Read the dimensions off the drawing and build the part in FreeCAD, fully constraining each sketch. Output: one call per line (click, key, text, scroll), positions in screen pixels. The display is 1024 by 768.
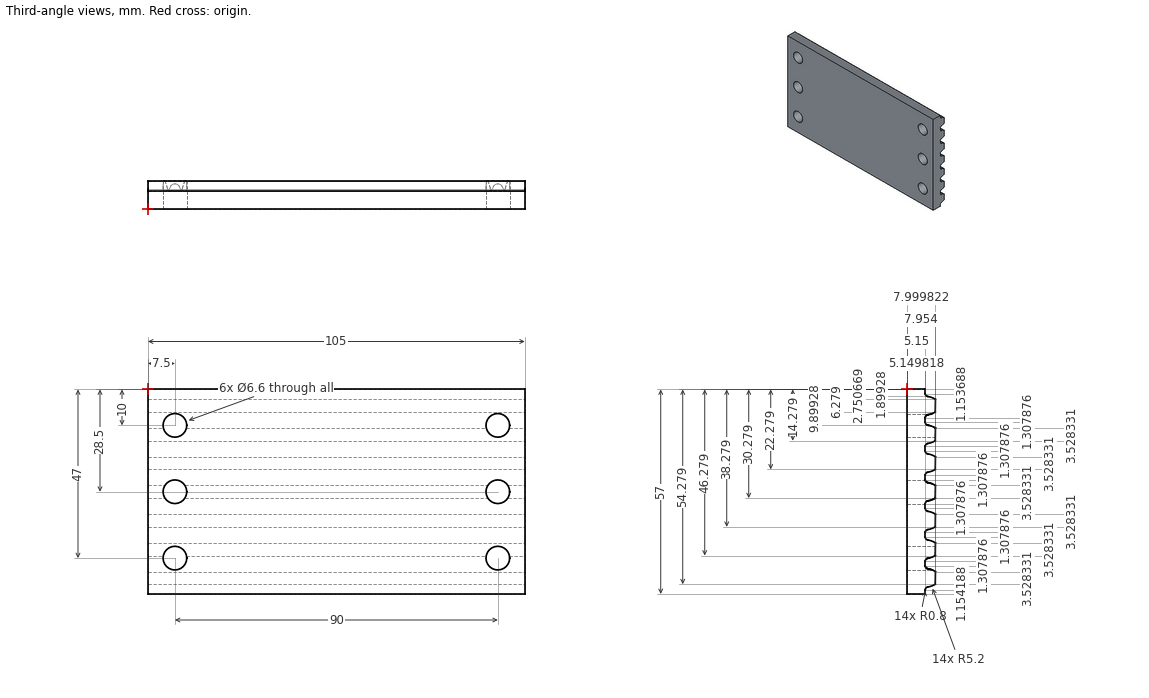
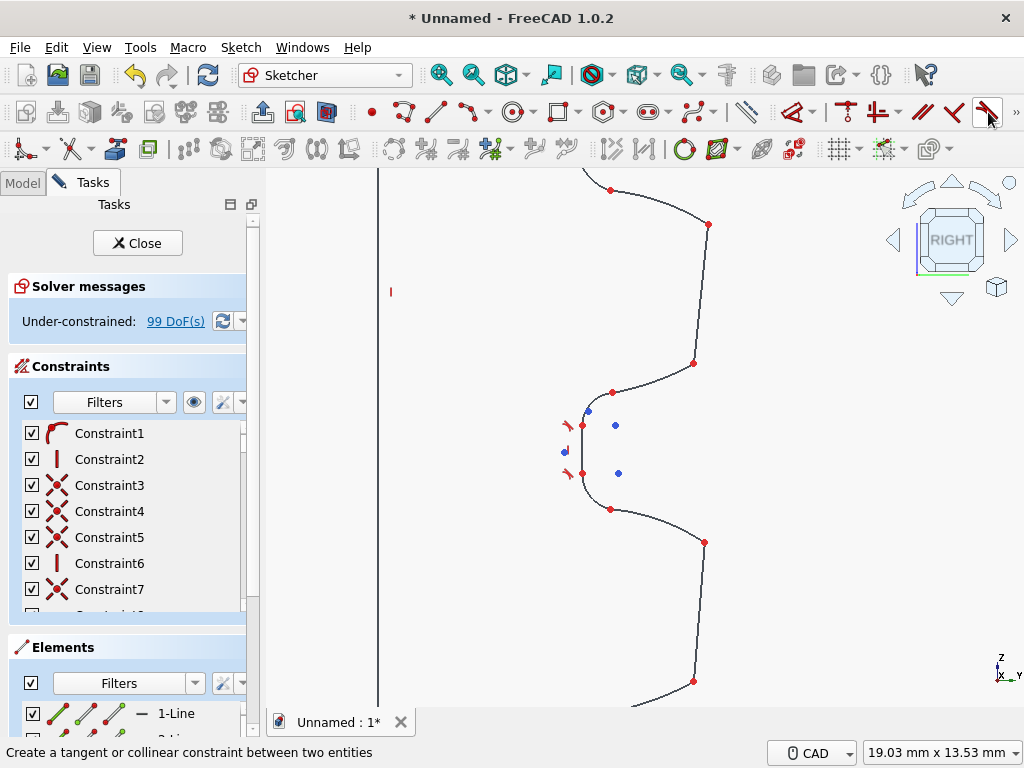
scroll(584, 467, down, 9)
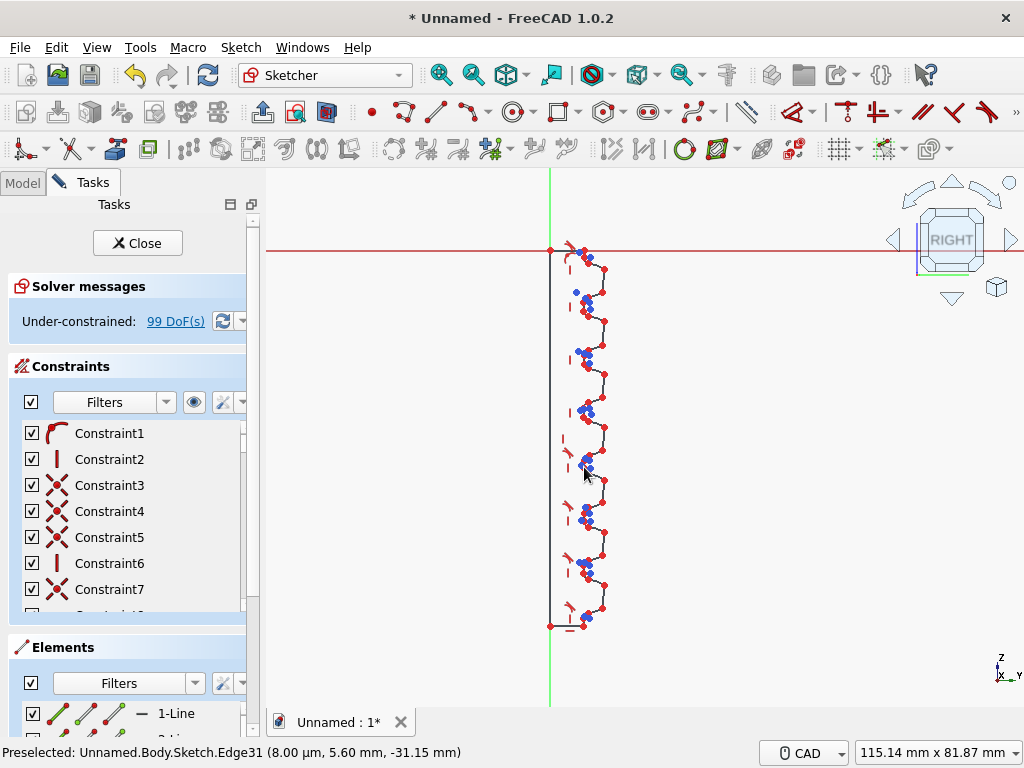
scroll(584, 415, up, 8)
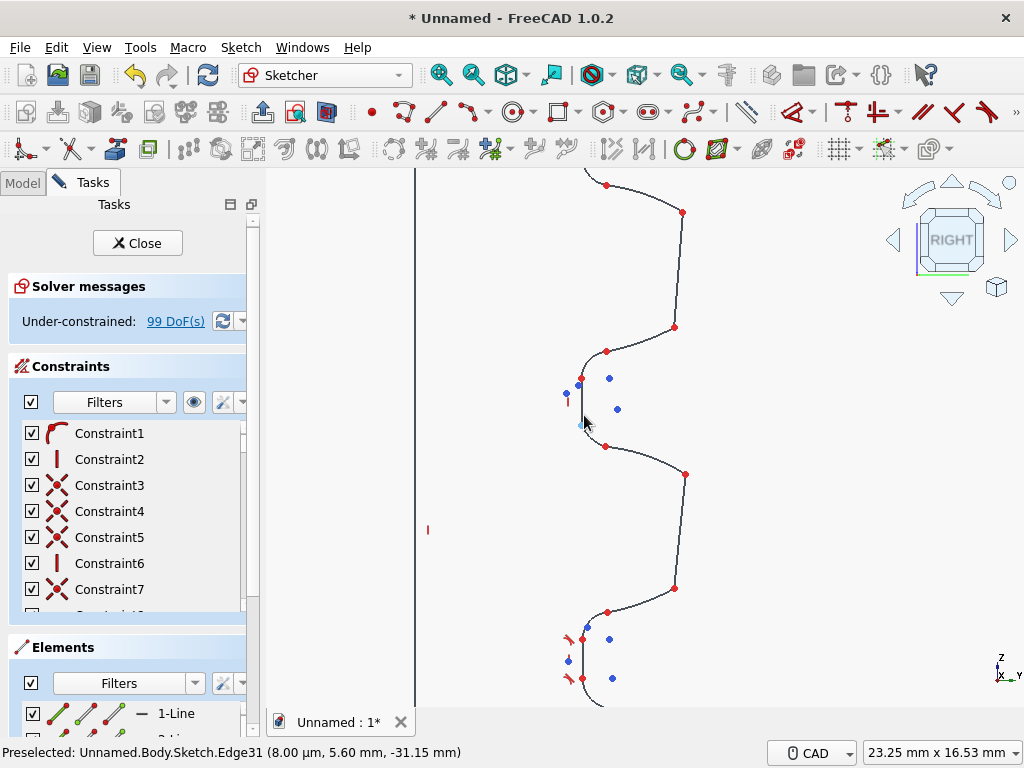
click(582, 411)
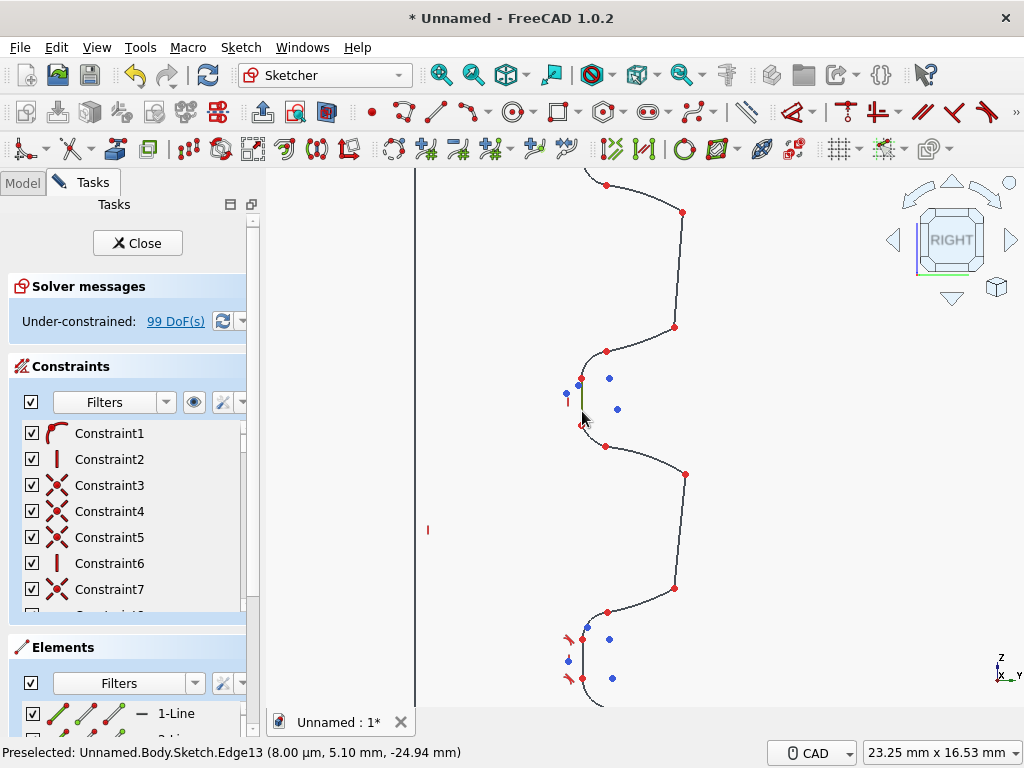
scroll(587, 434, up, 2)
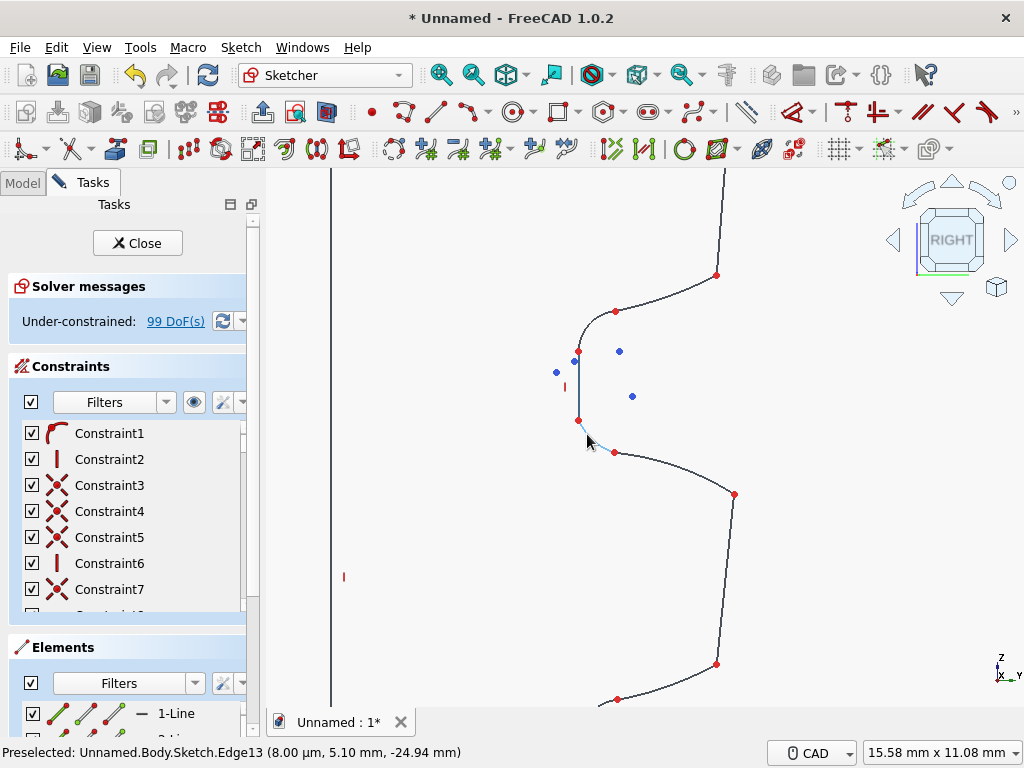
click(586, 433)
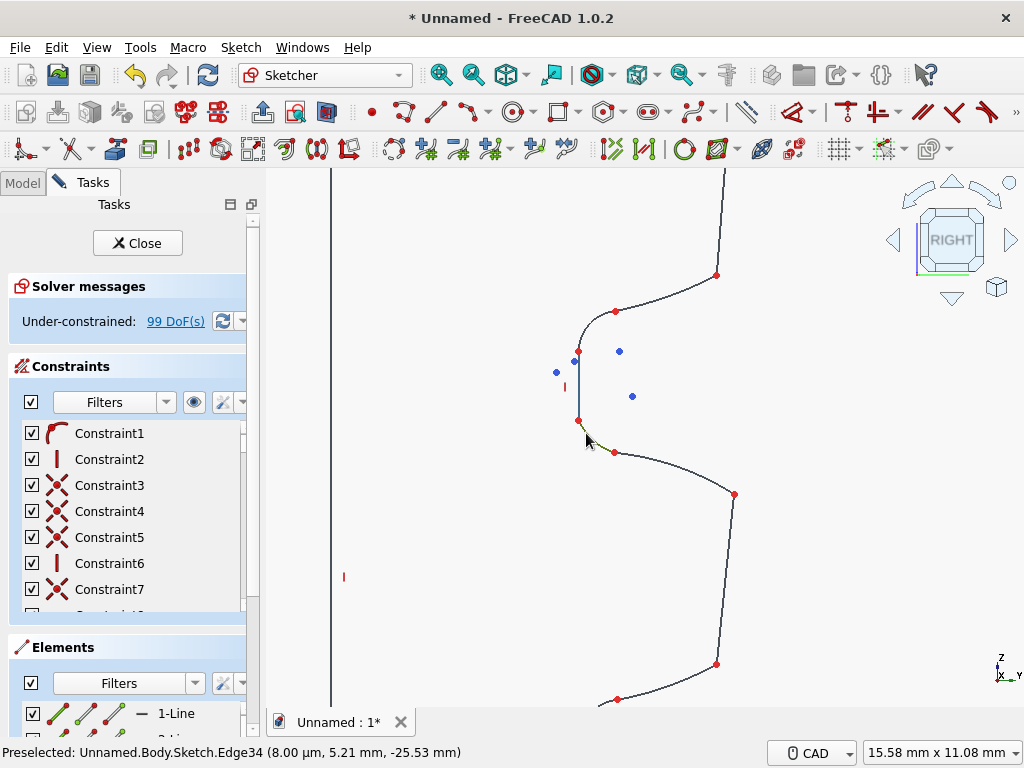
click(988, 112)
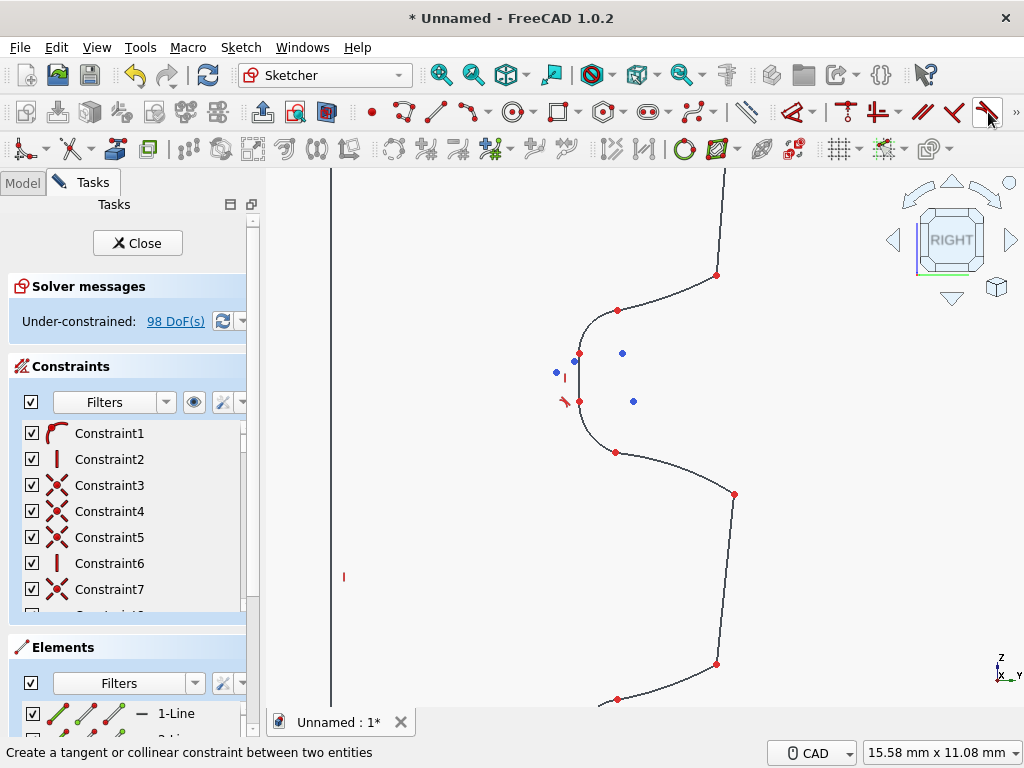
click(579, 387)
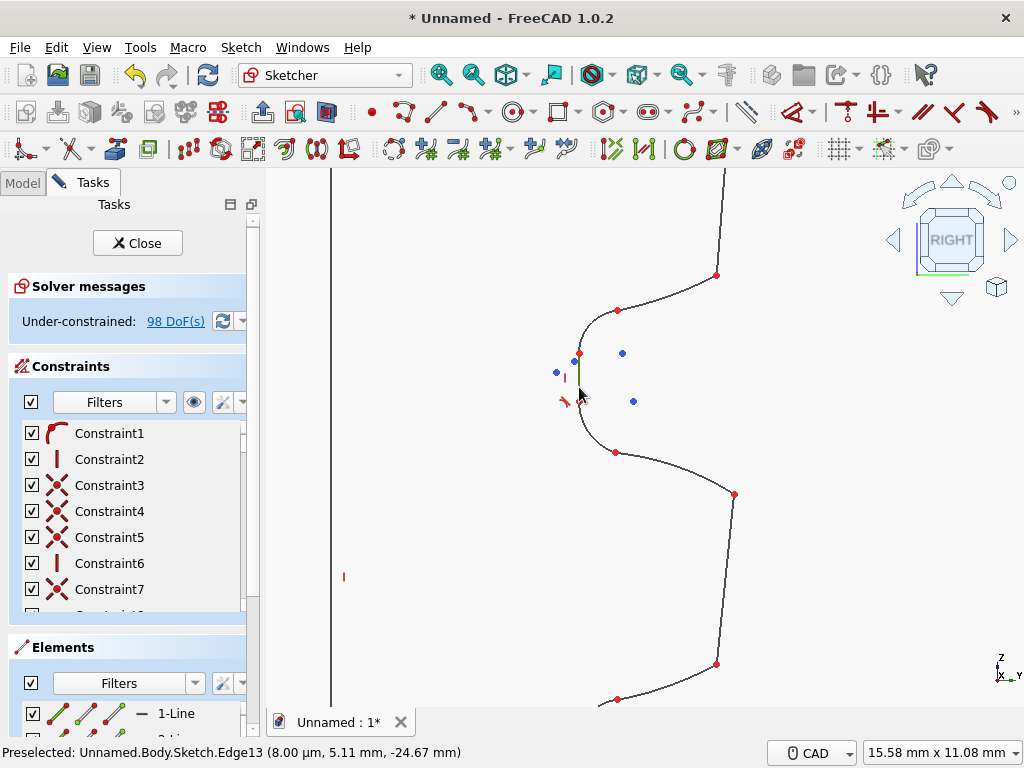
click(600, 317)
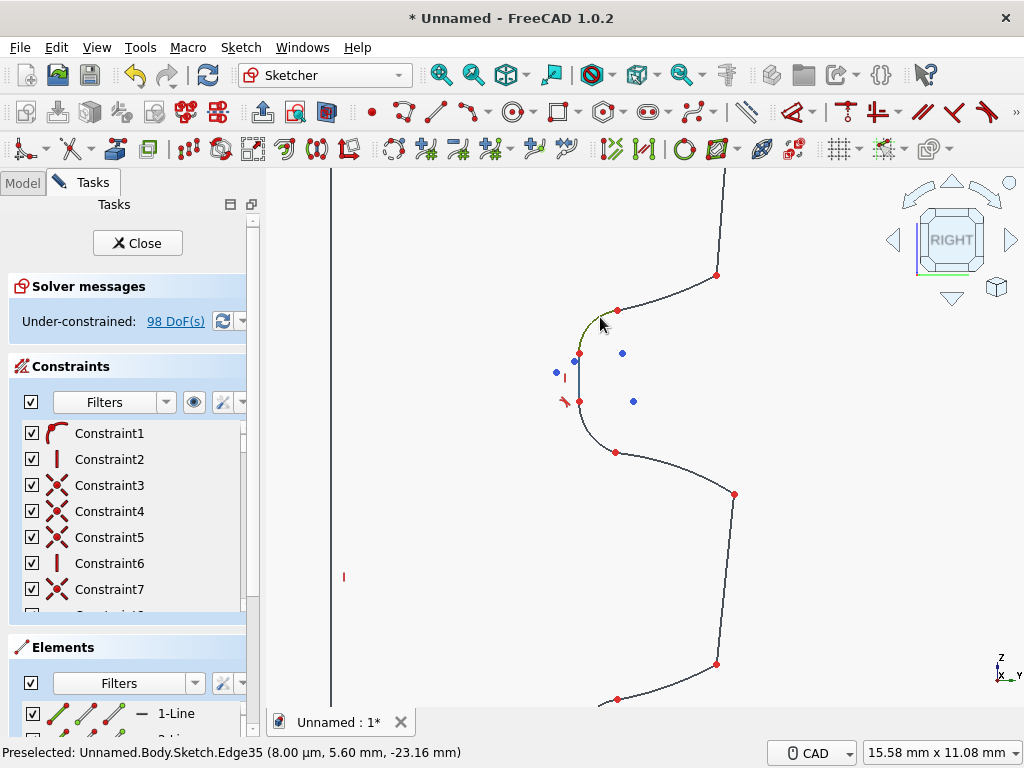
click(988, 112)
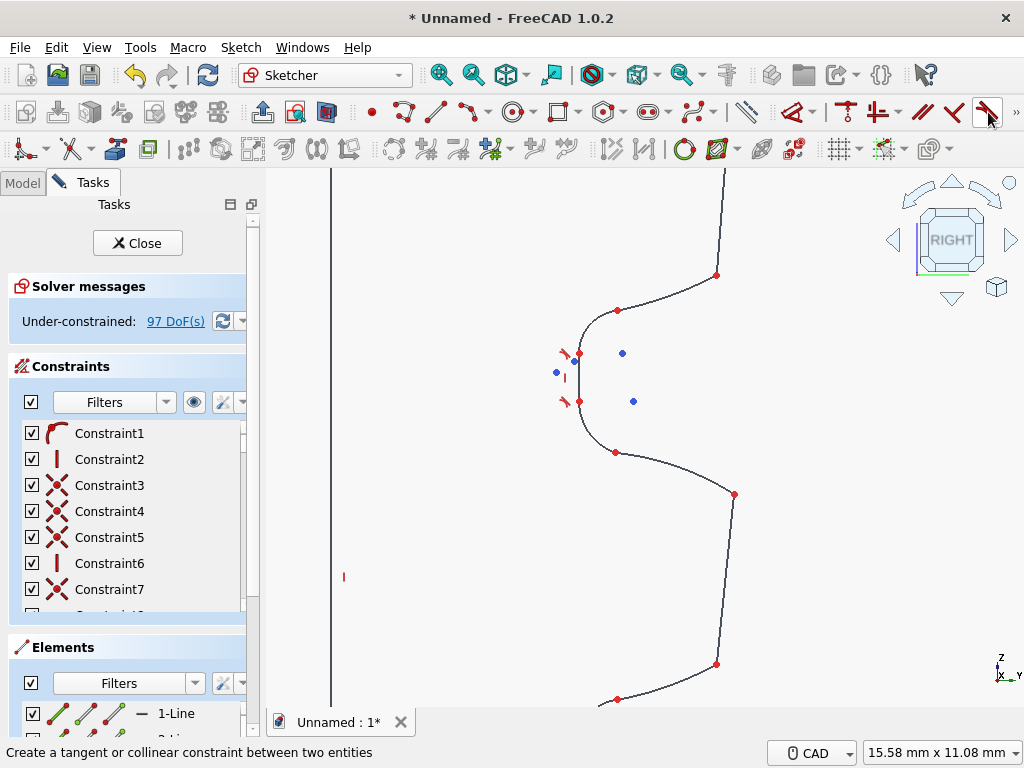
scroll(585, 416, down, 10)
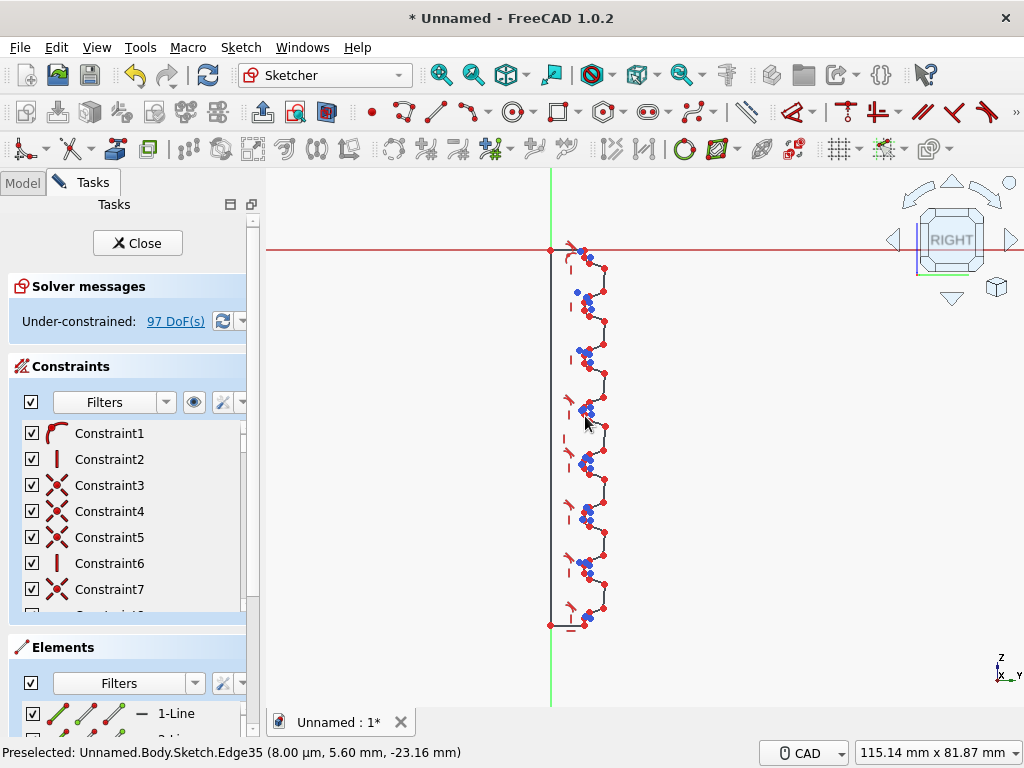
scroll(585, 361, up, 9)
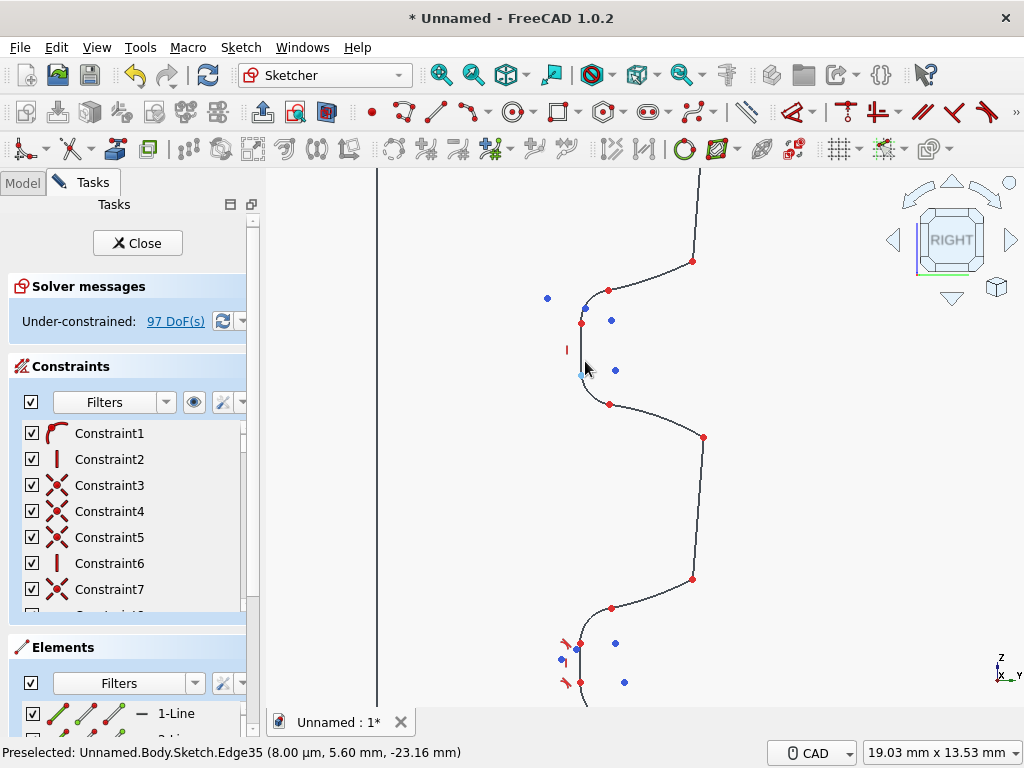
click(581, 360)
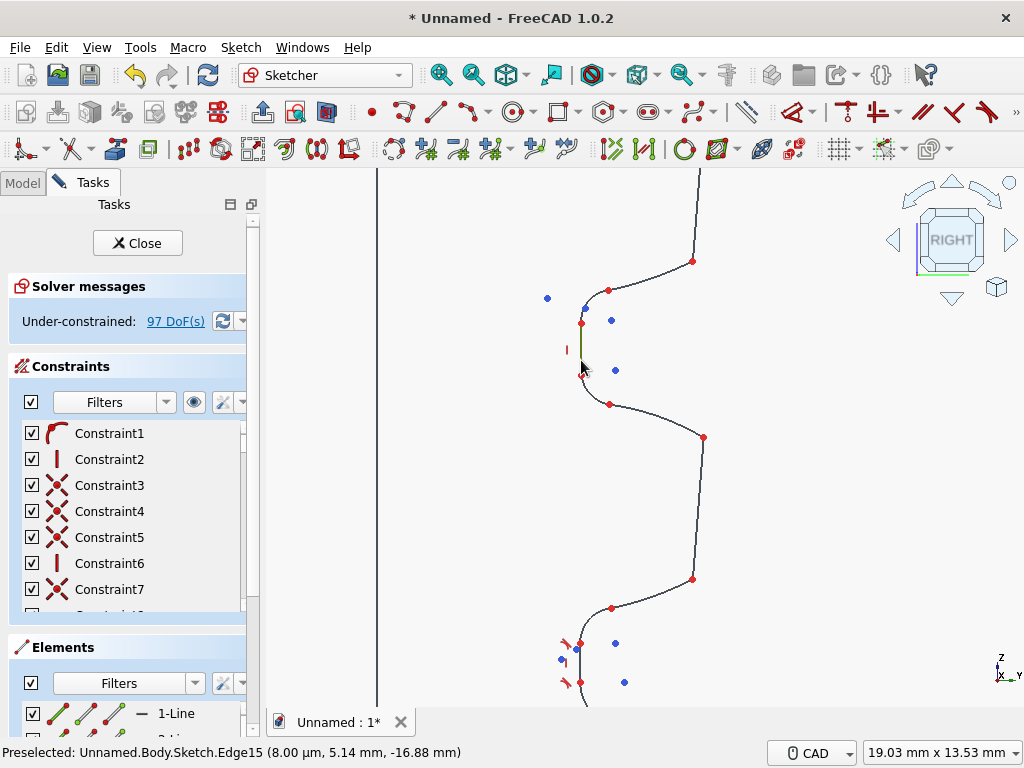
click(586, 388)